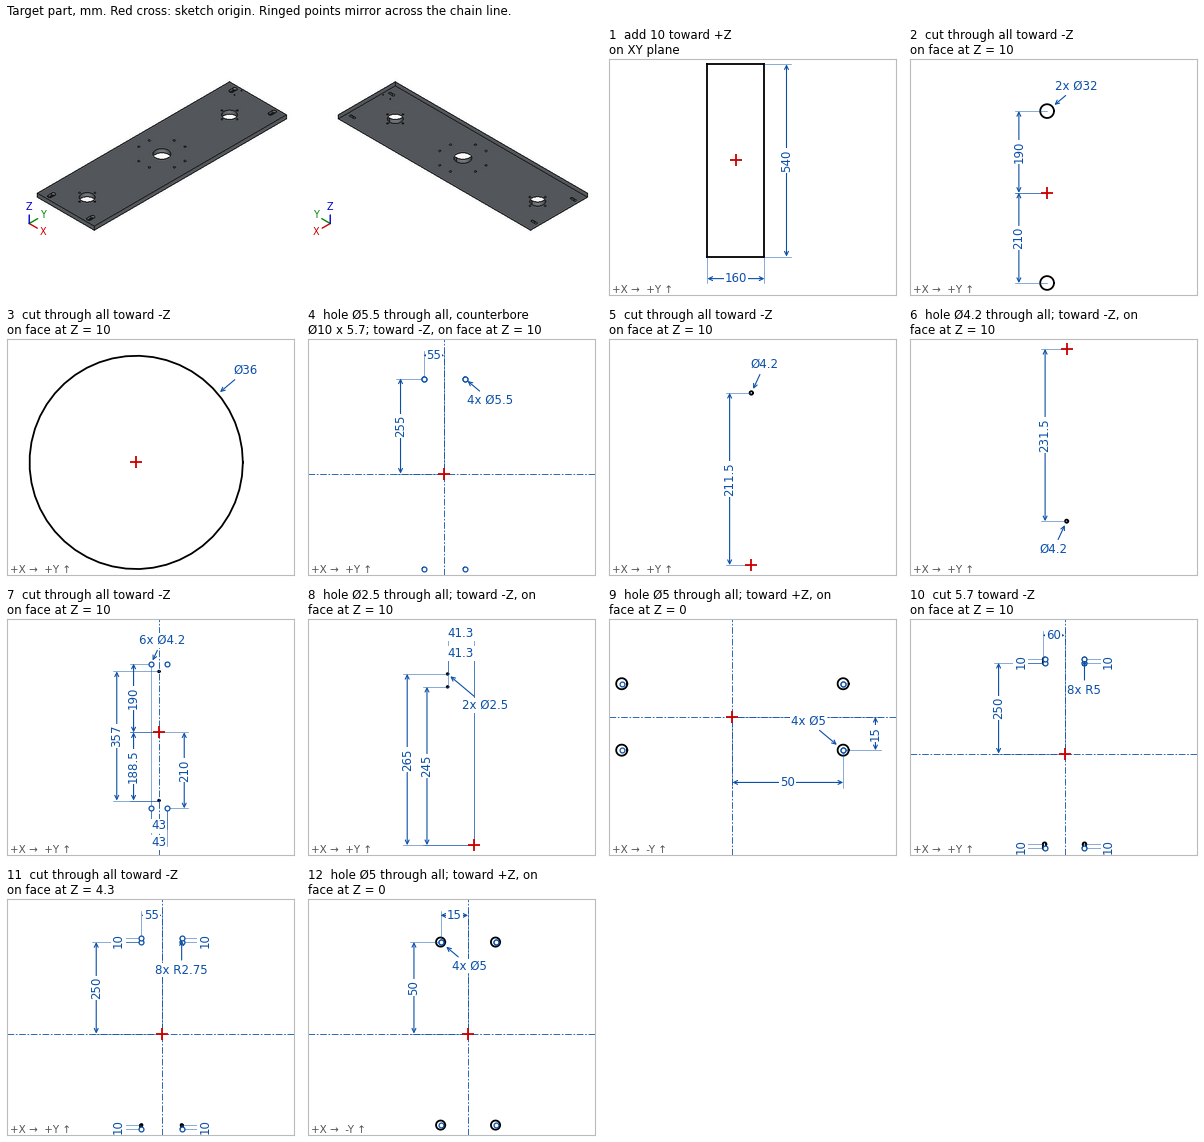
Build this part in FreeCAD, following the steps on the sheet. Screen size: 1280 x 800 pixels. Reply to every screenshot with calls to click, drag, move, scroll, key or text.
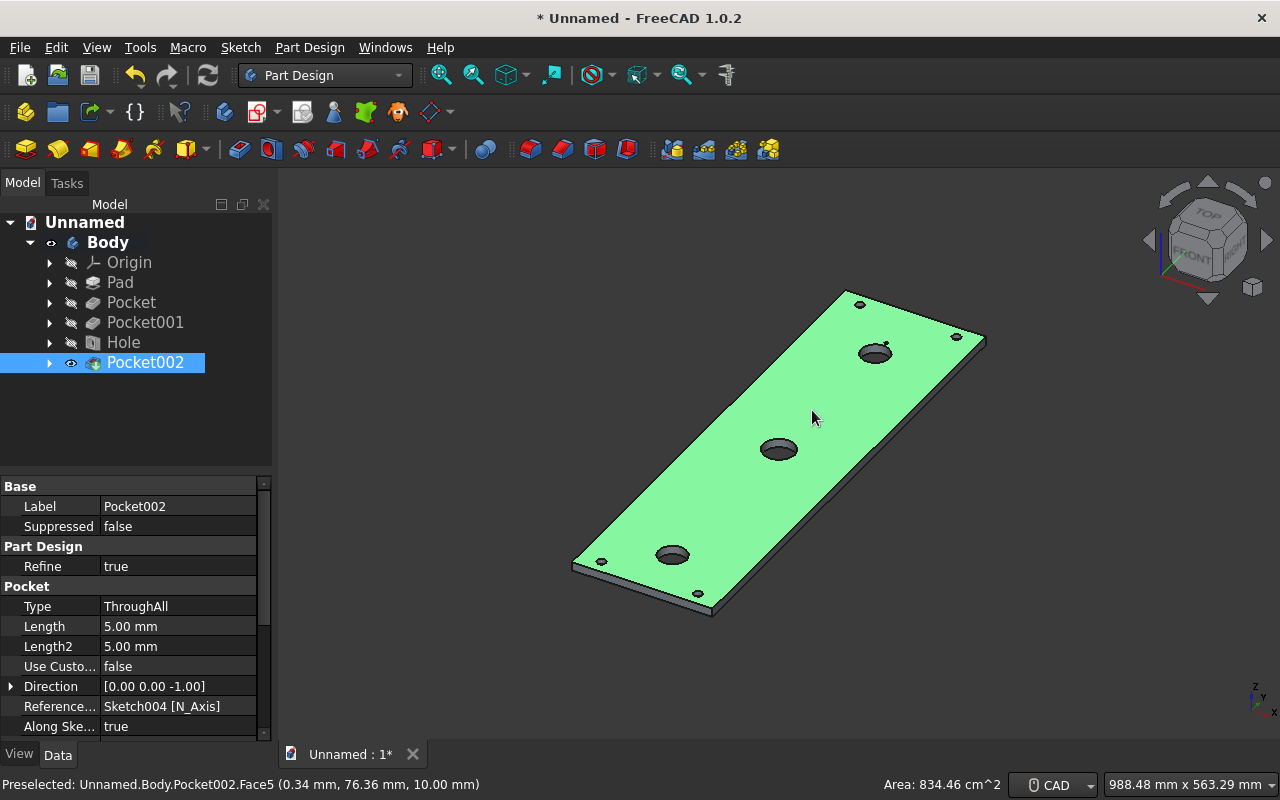
click(258, 112)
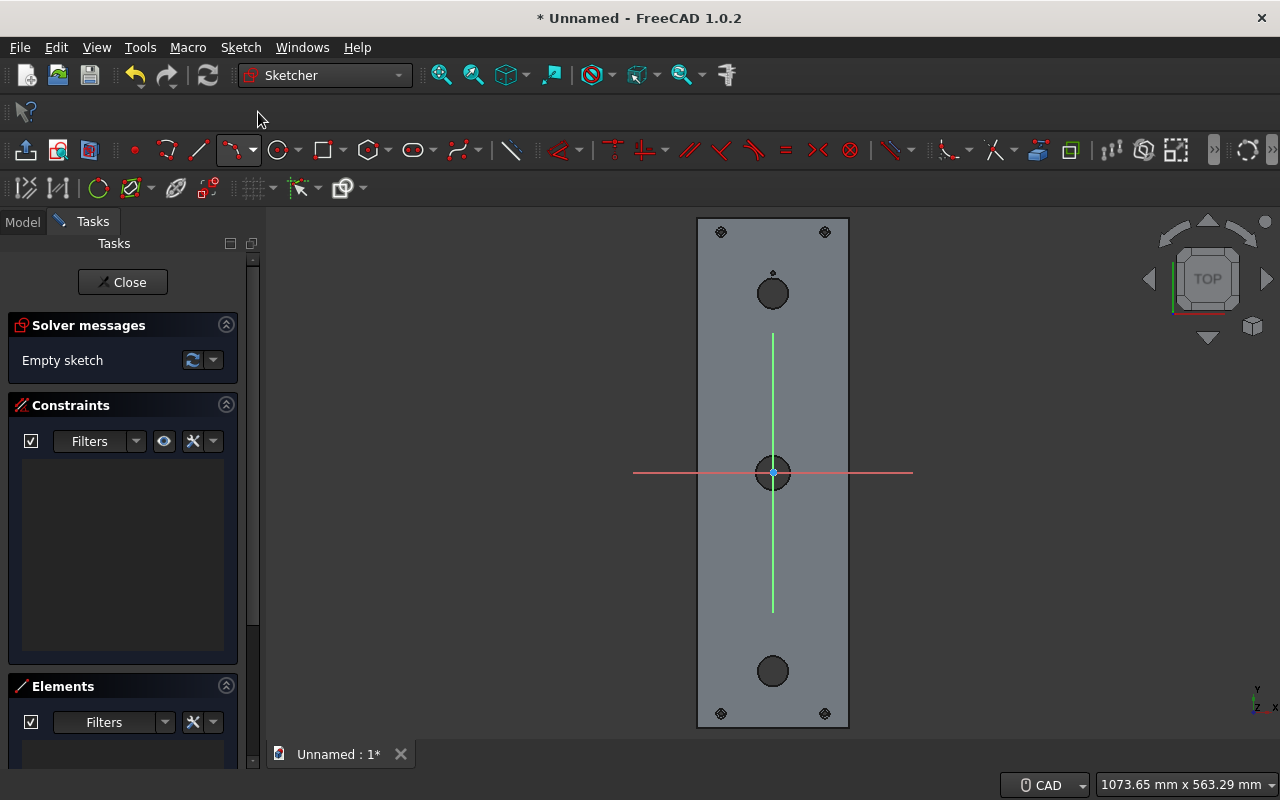
scroll(777, 703, up, 15)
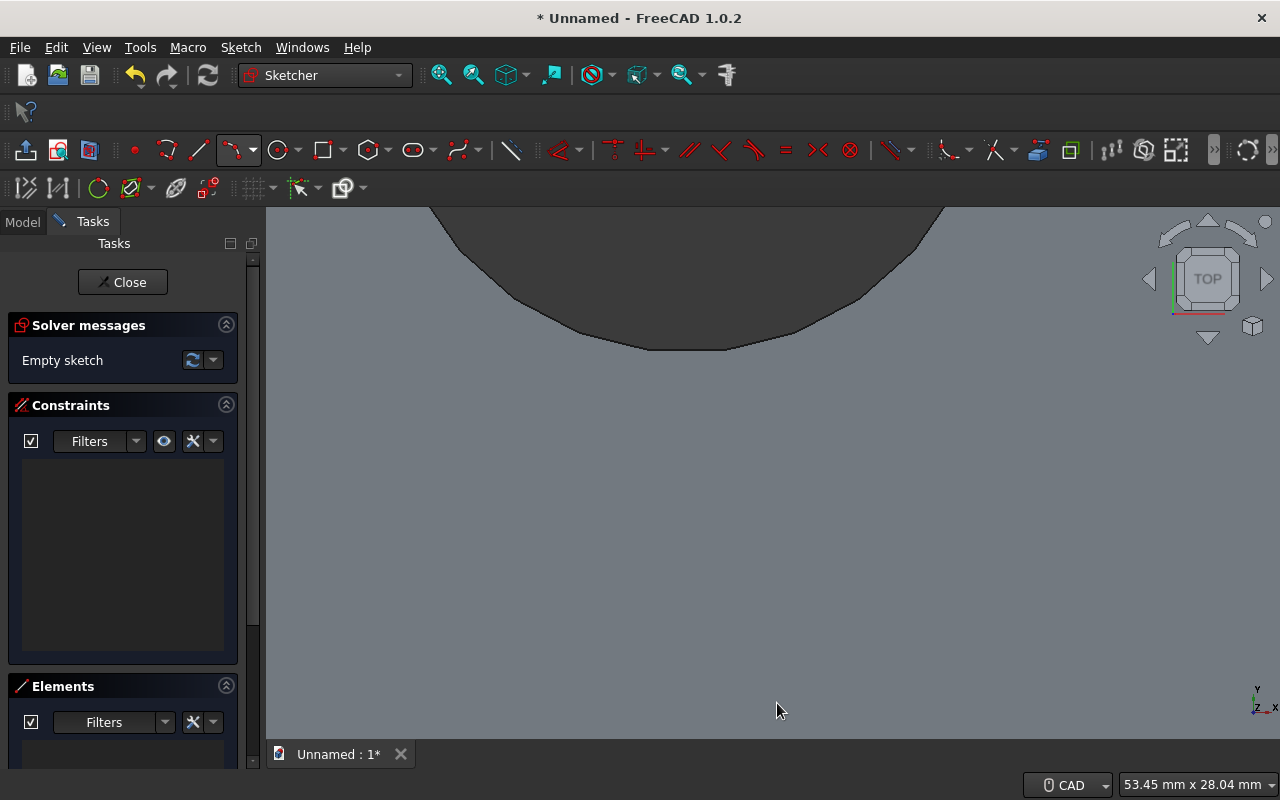
scroll(681, 452, up, 7)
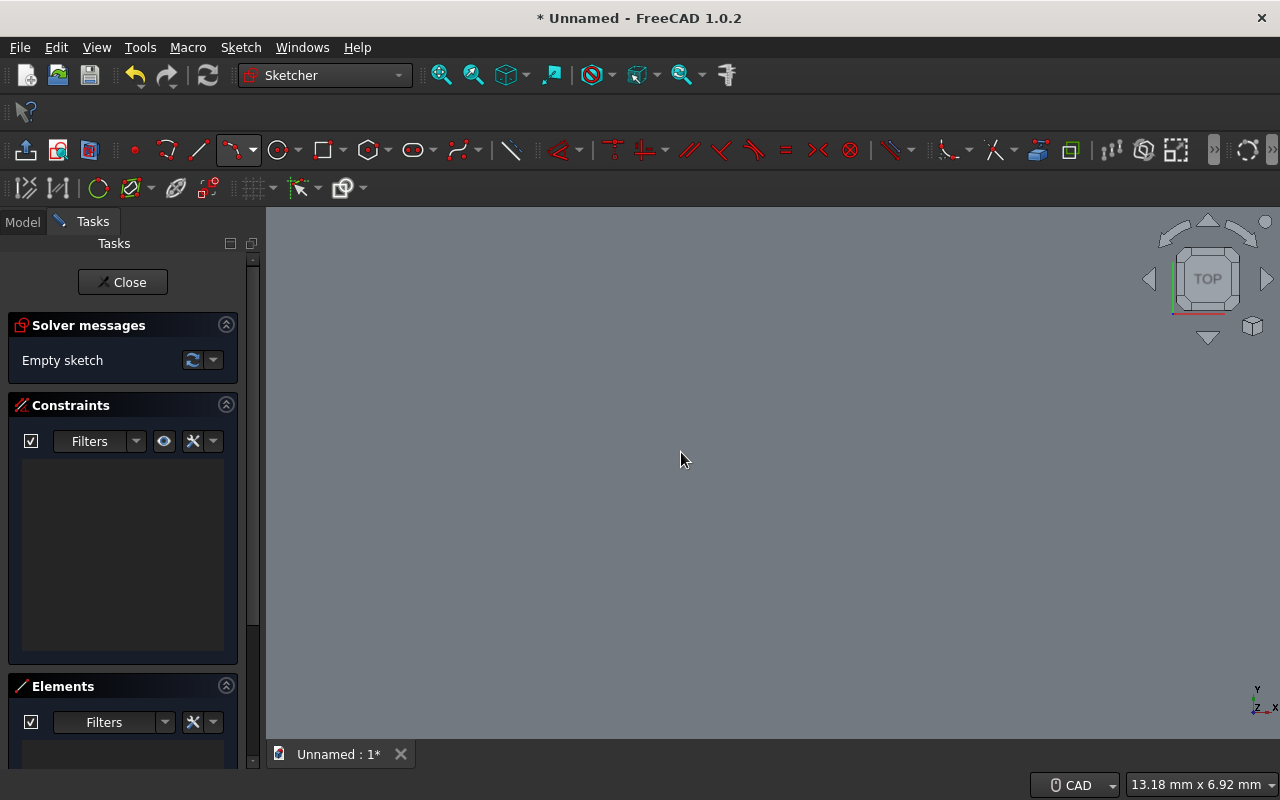
key(g)
key(c)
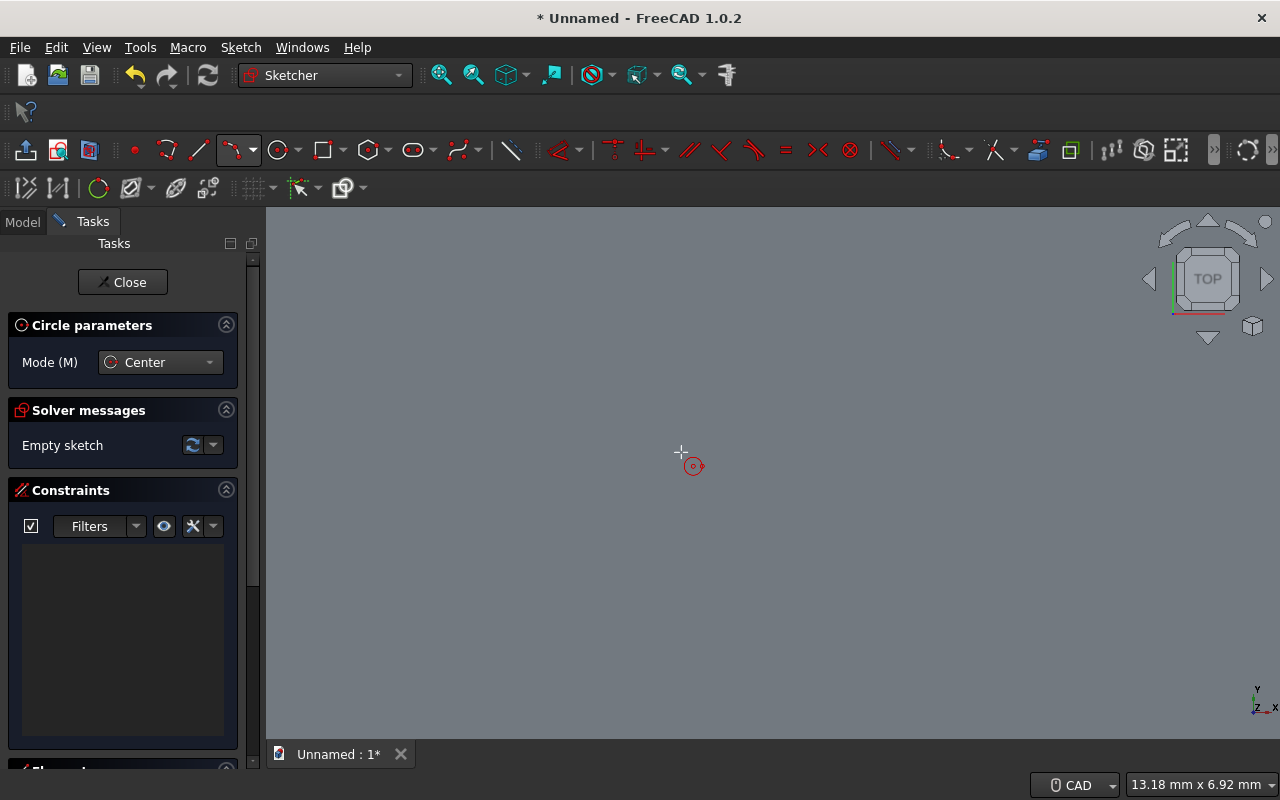
click(704, 471)
move(818, 357)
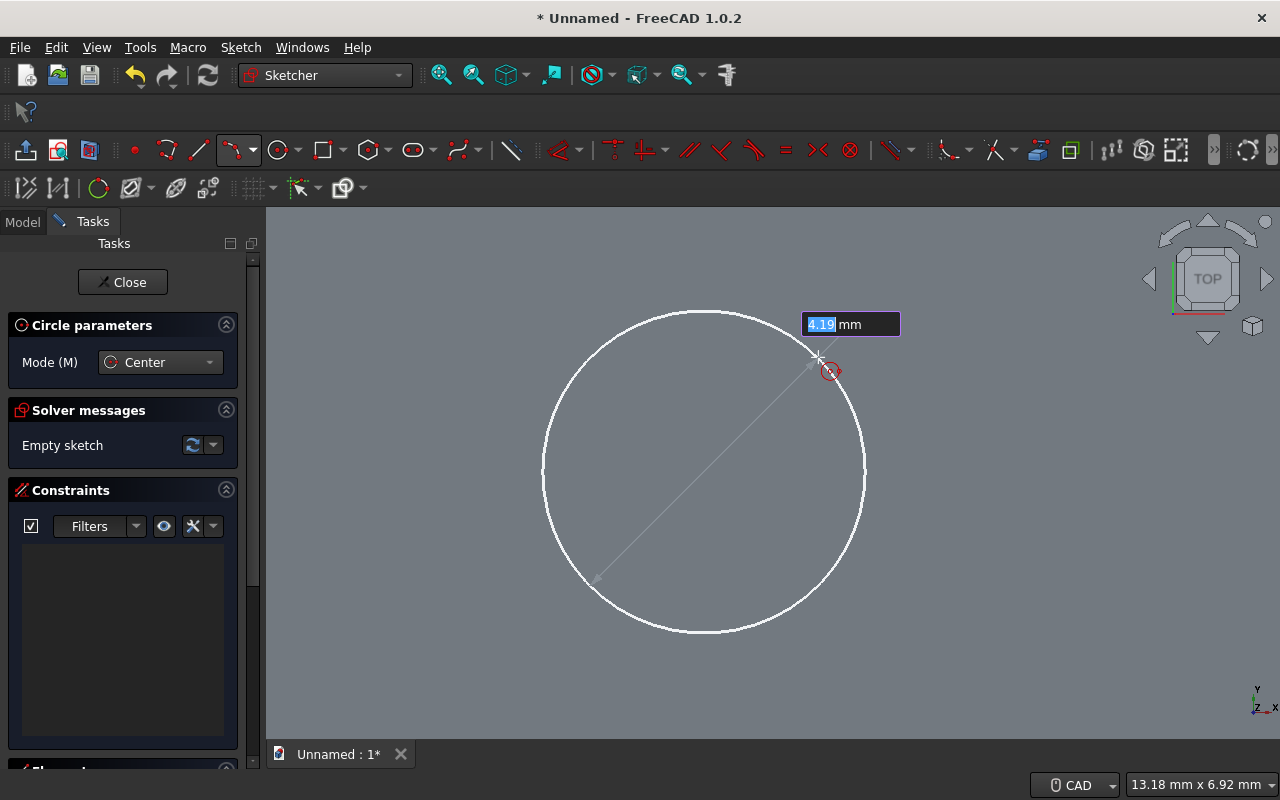
text(4.2)
key(Return)
key(Escape)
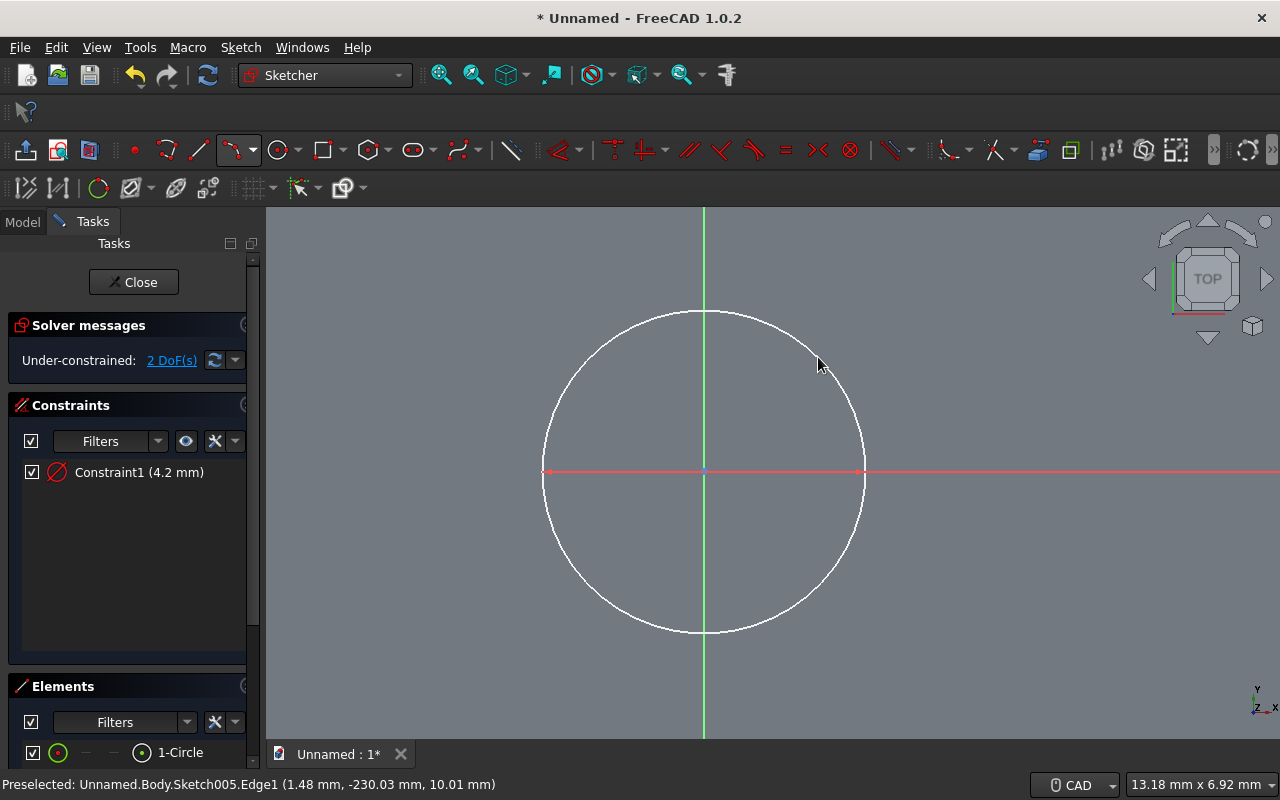
click(704, 472)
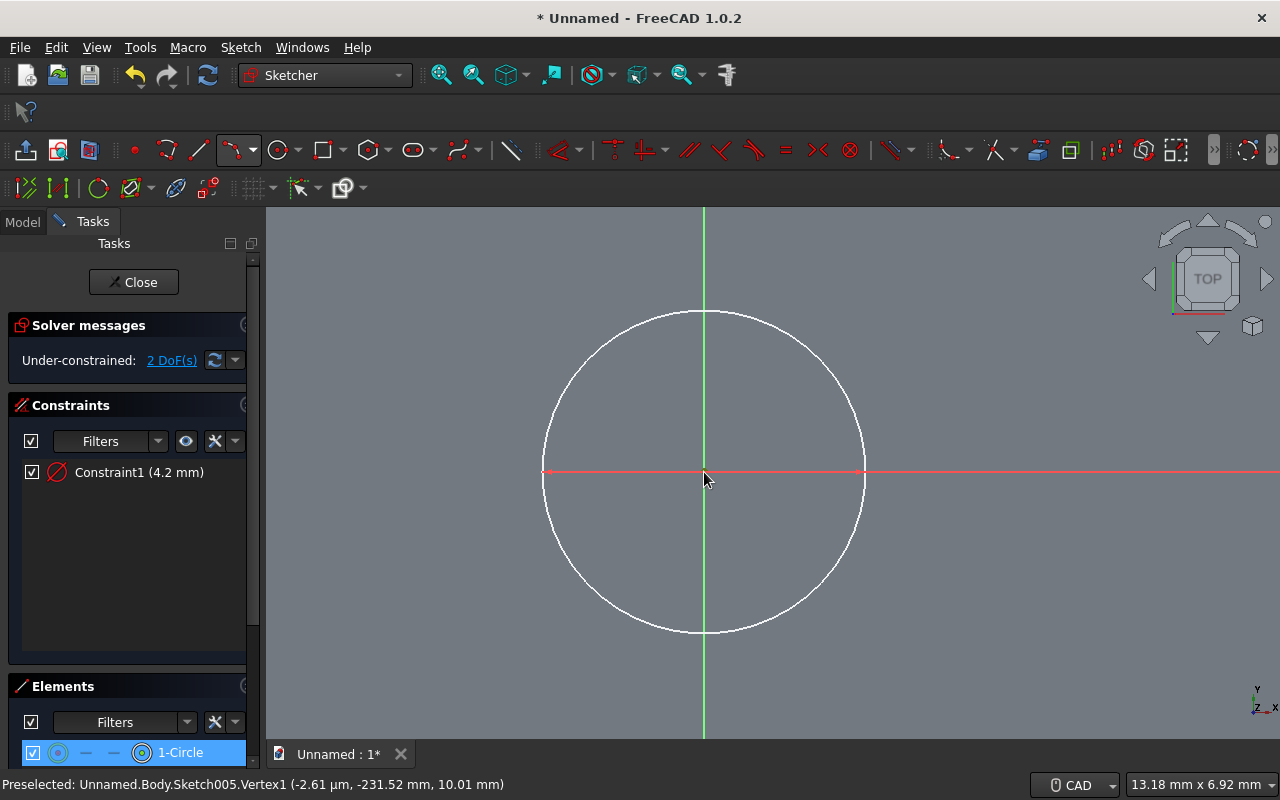
click(704, 677)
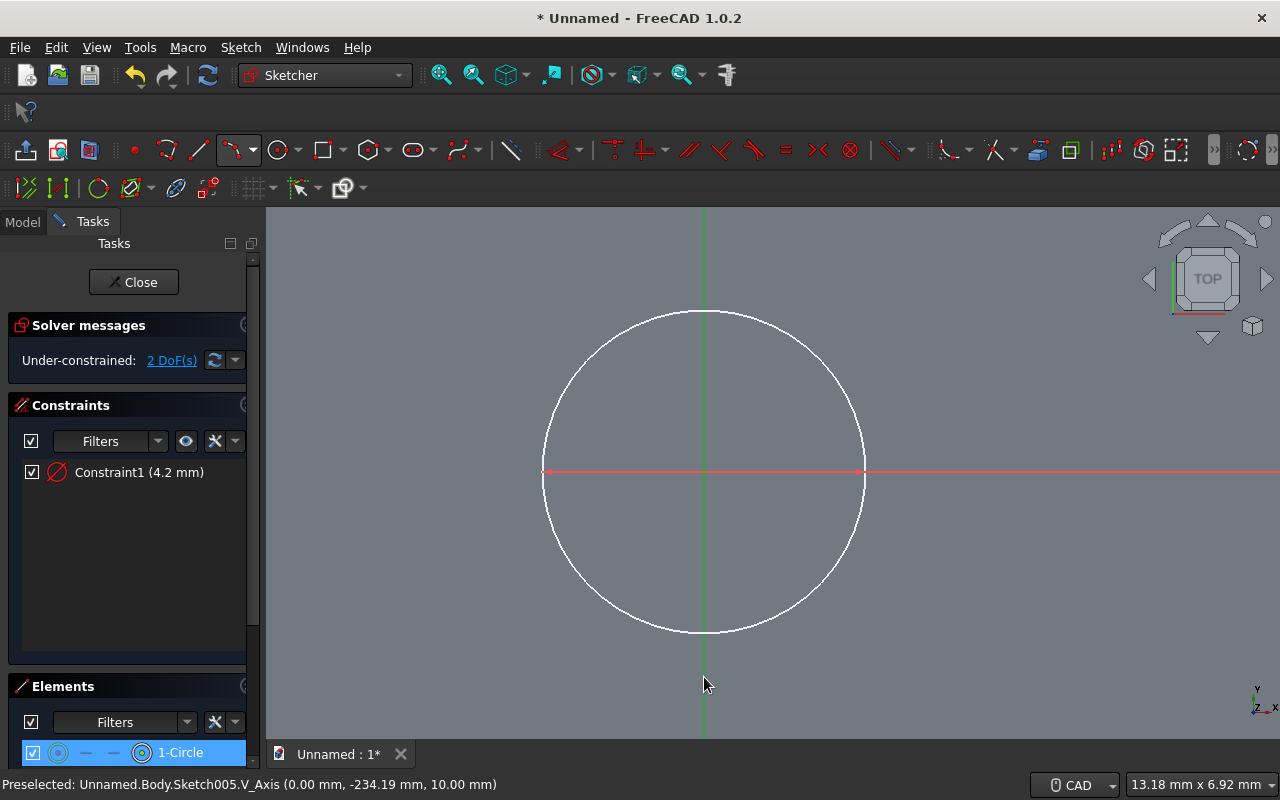
key(c)